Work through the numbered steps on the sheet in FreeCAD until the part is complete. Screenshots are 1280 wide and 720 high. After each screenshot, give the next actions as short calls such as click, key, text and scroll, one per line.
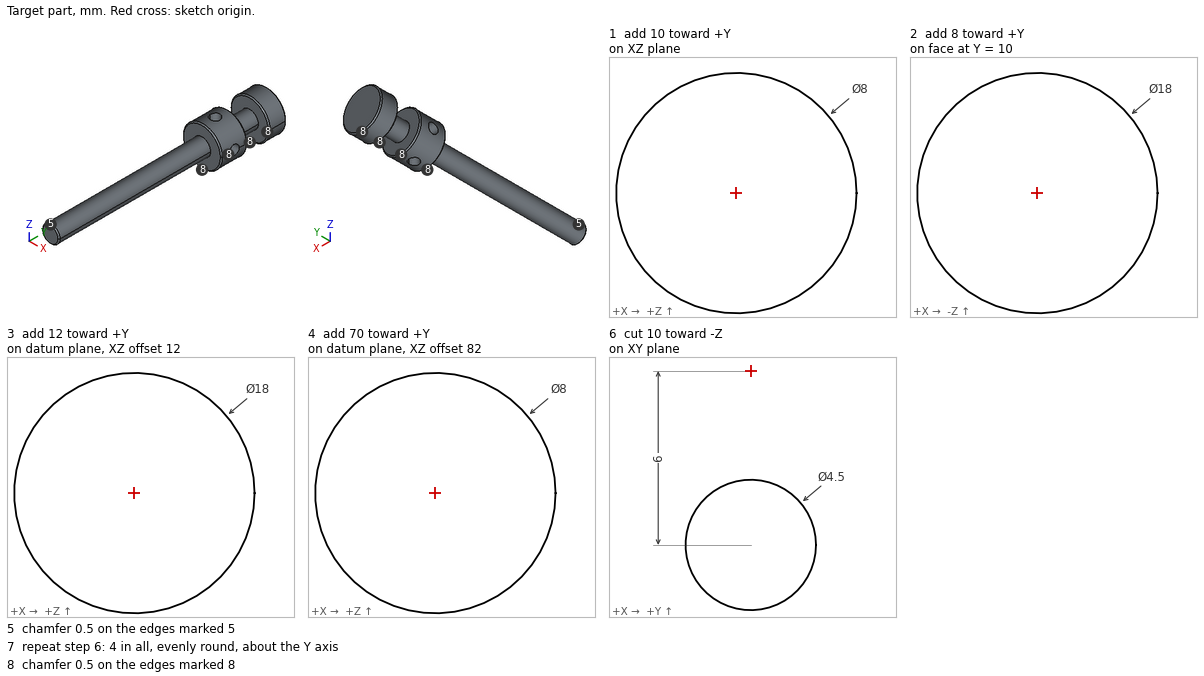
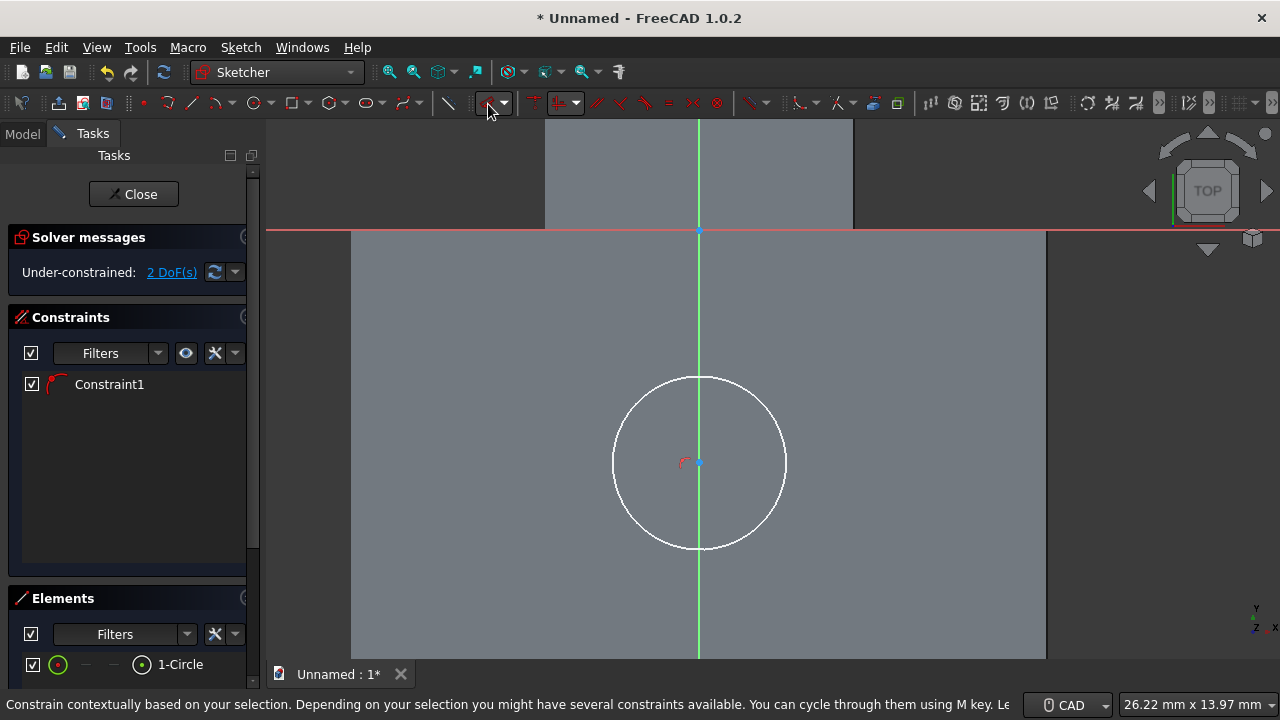
click(761, 402)
click(784, 379)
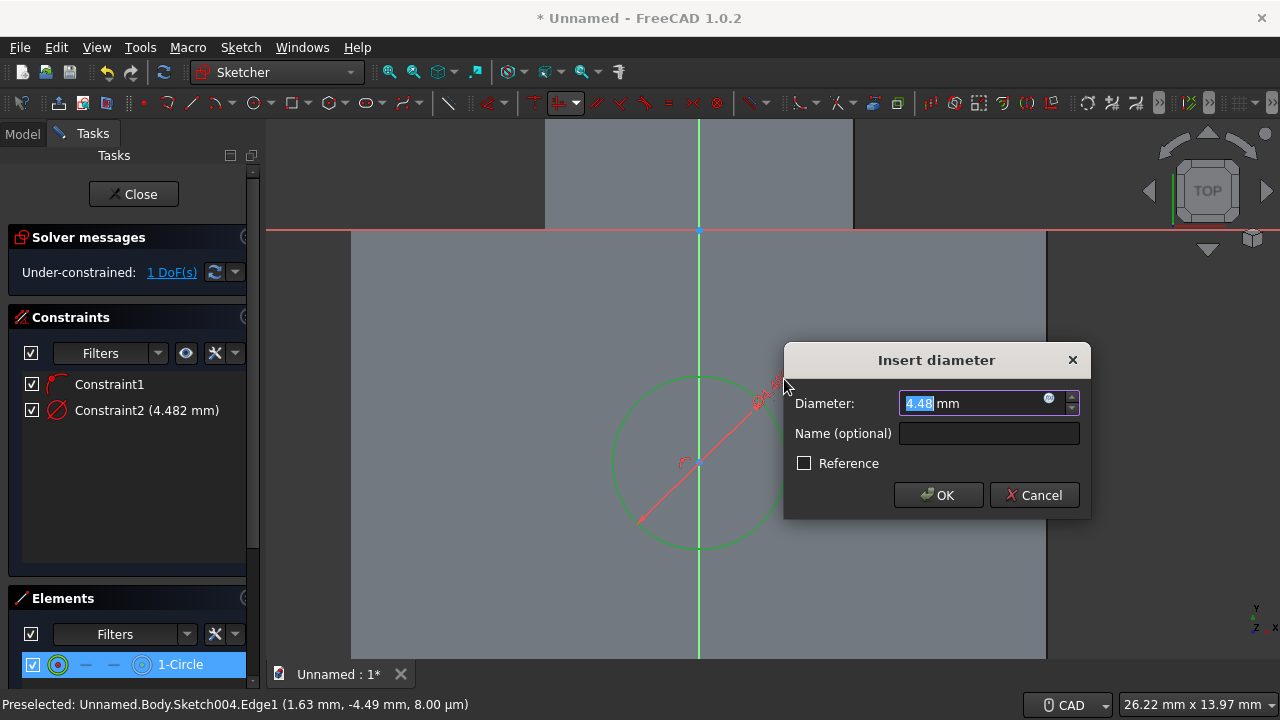
text(4.5)
key(Return)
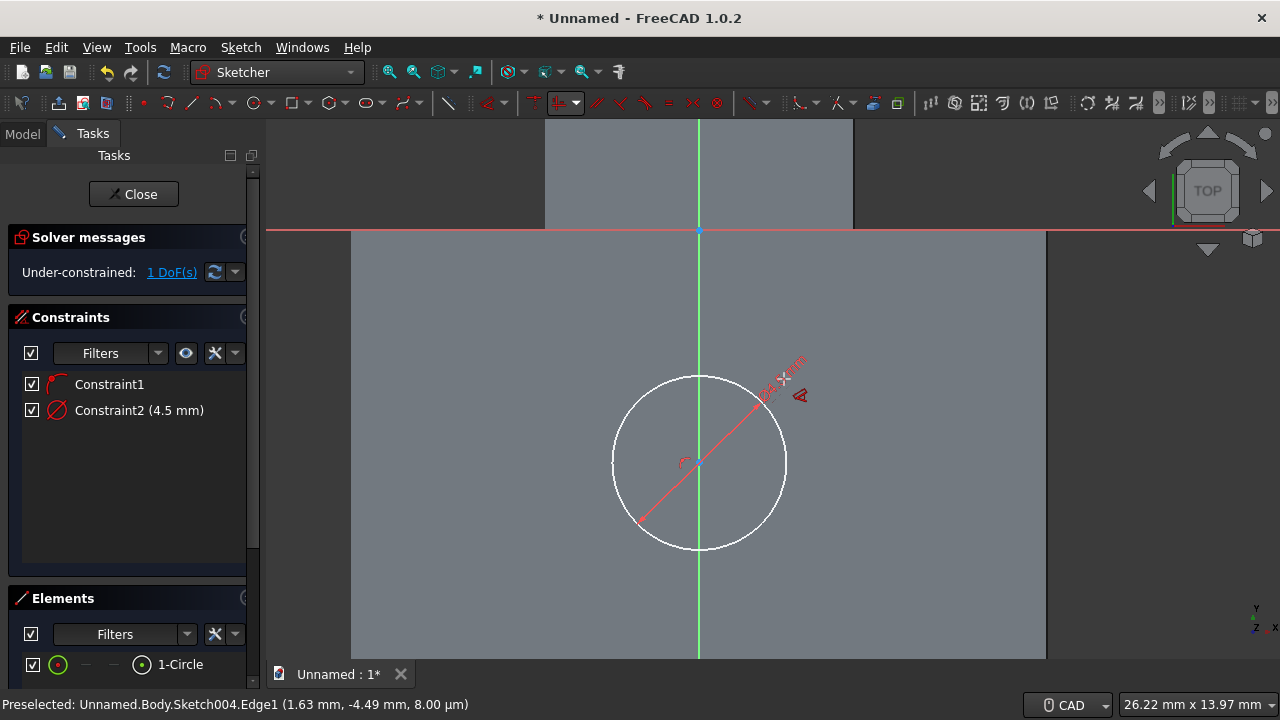
click(699, 463)
click(733, 347)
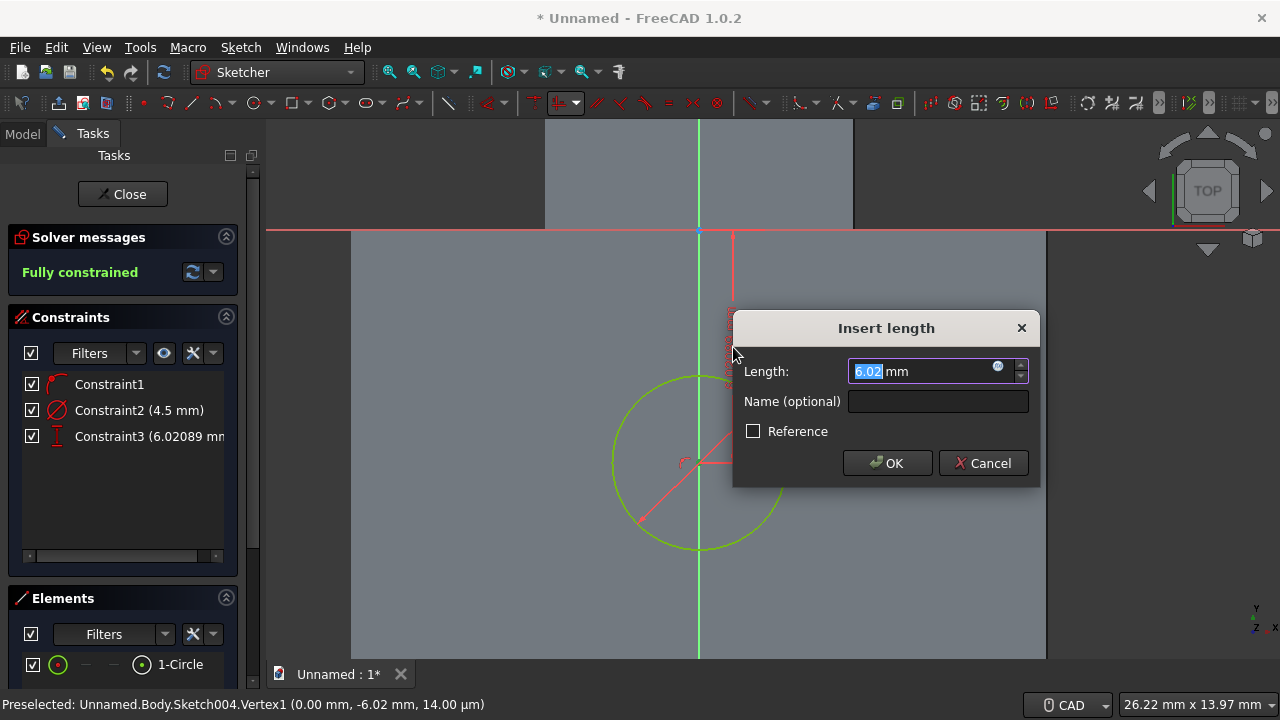
text(6)
key(Return)
key(Escape)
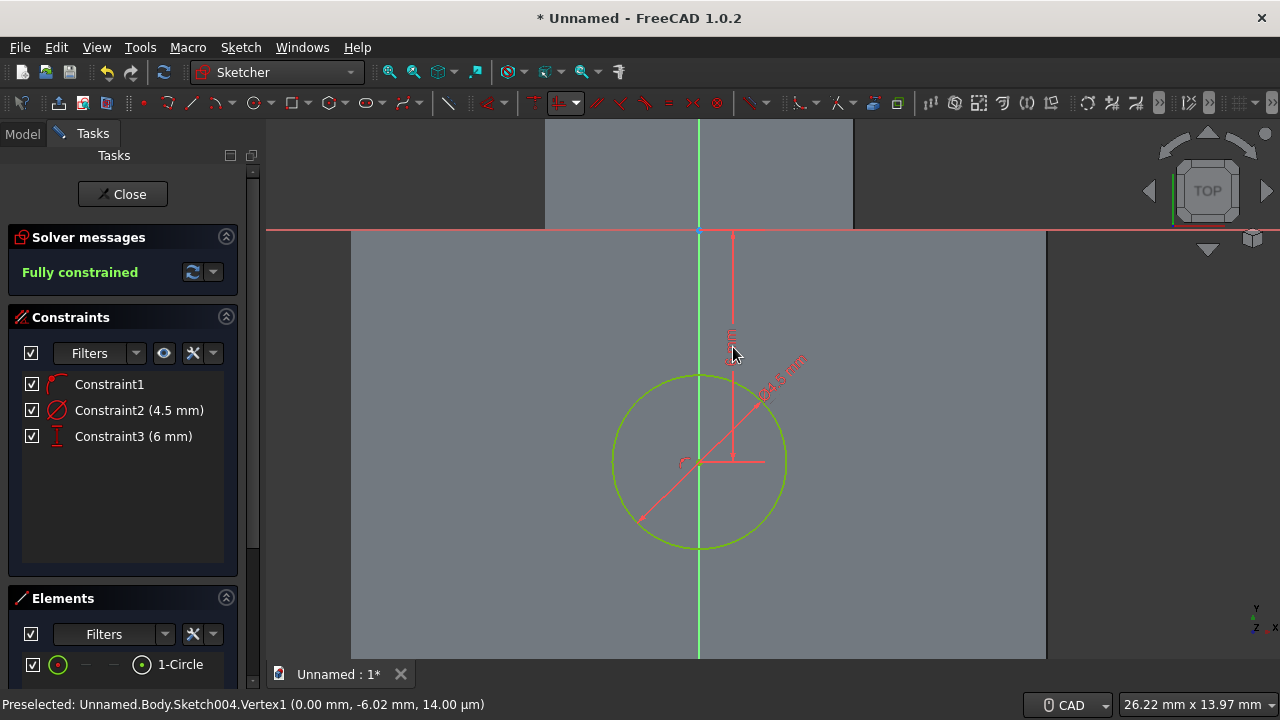
click(123, 194)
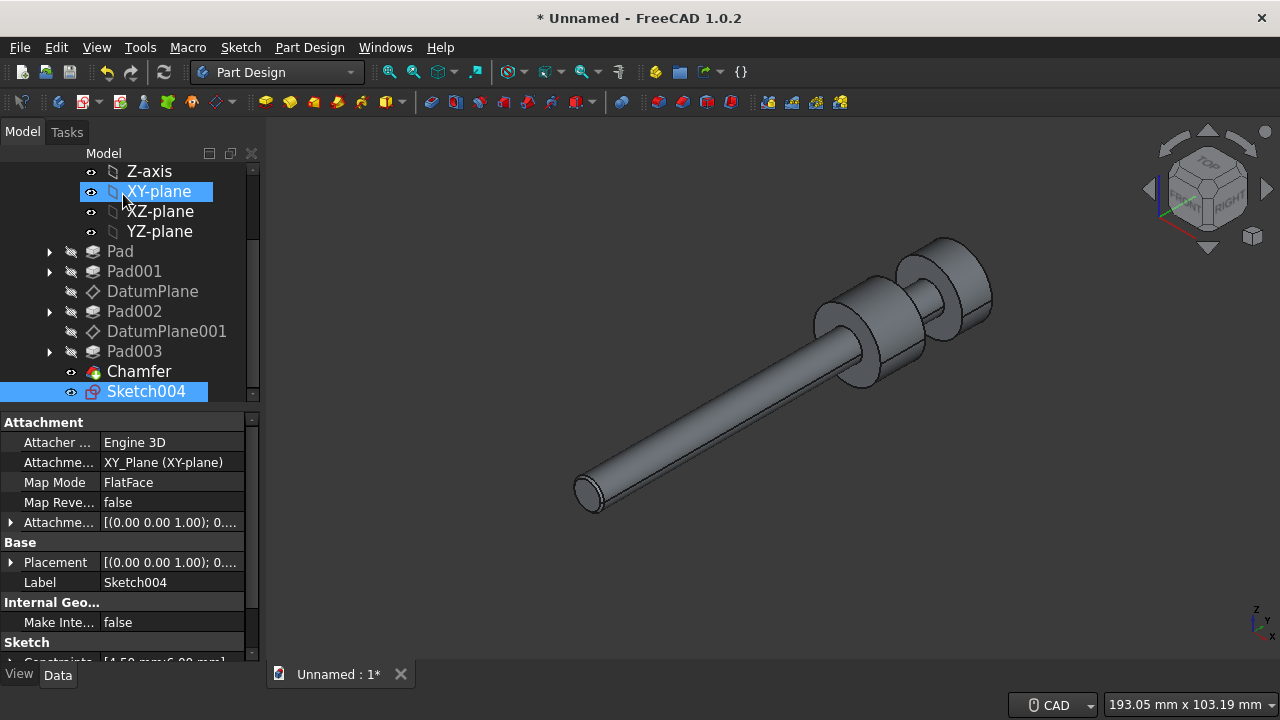
click(432, 102)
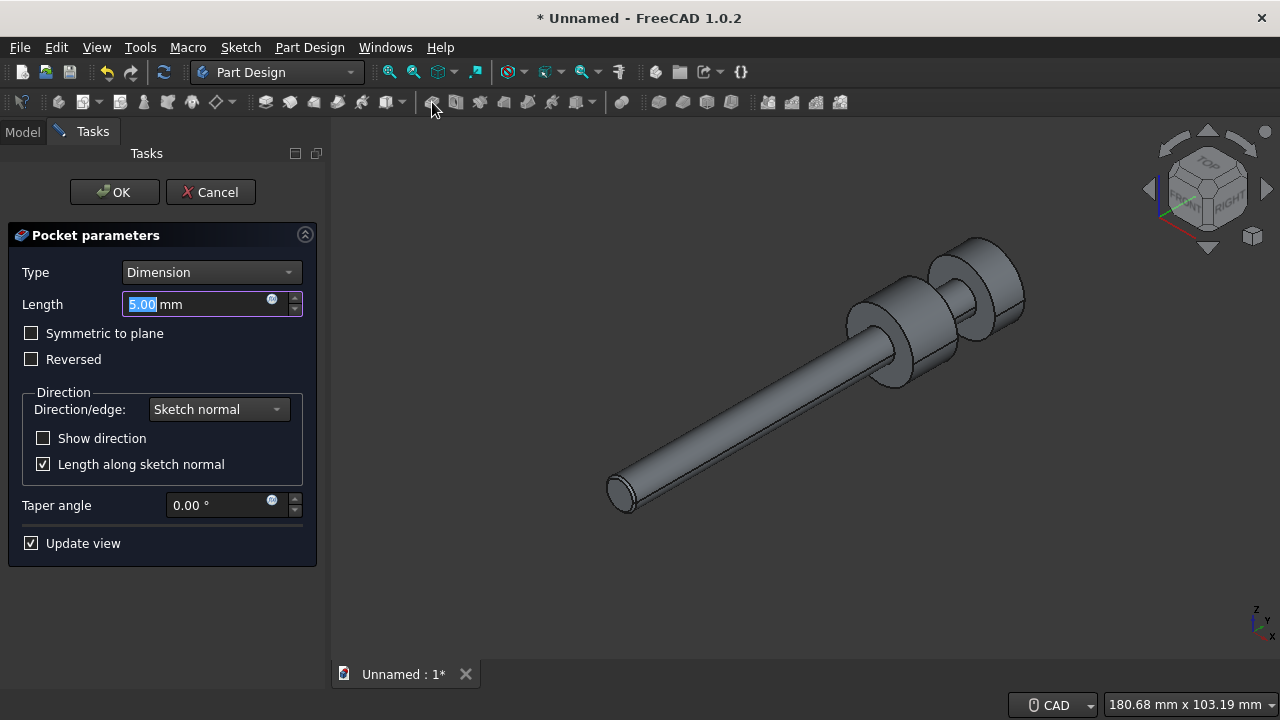
text(10)
key(Tab)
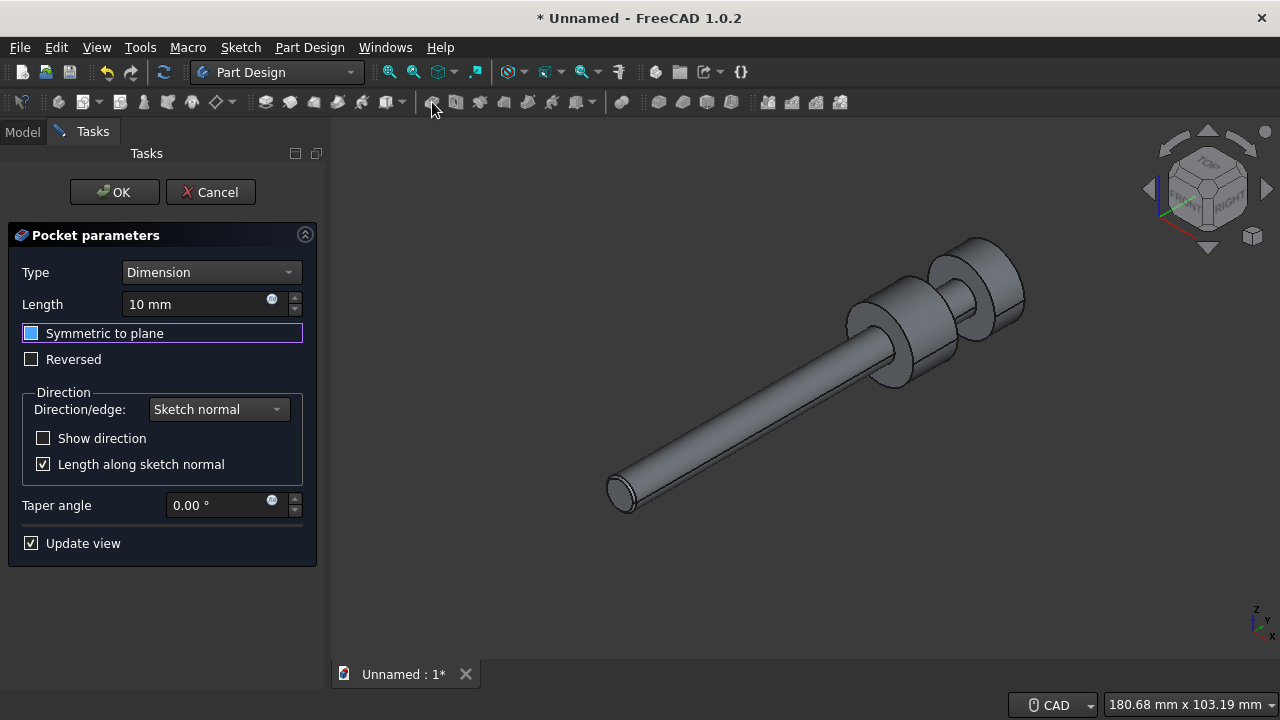
click(115, 192)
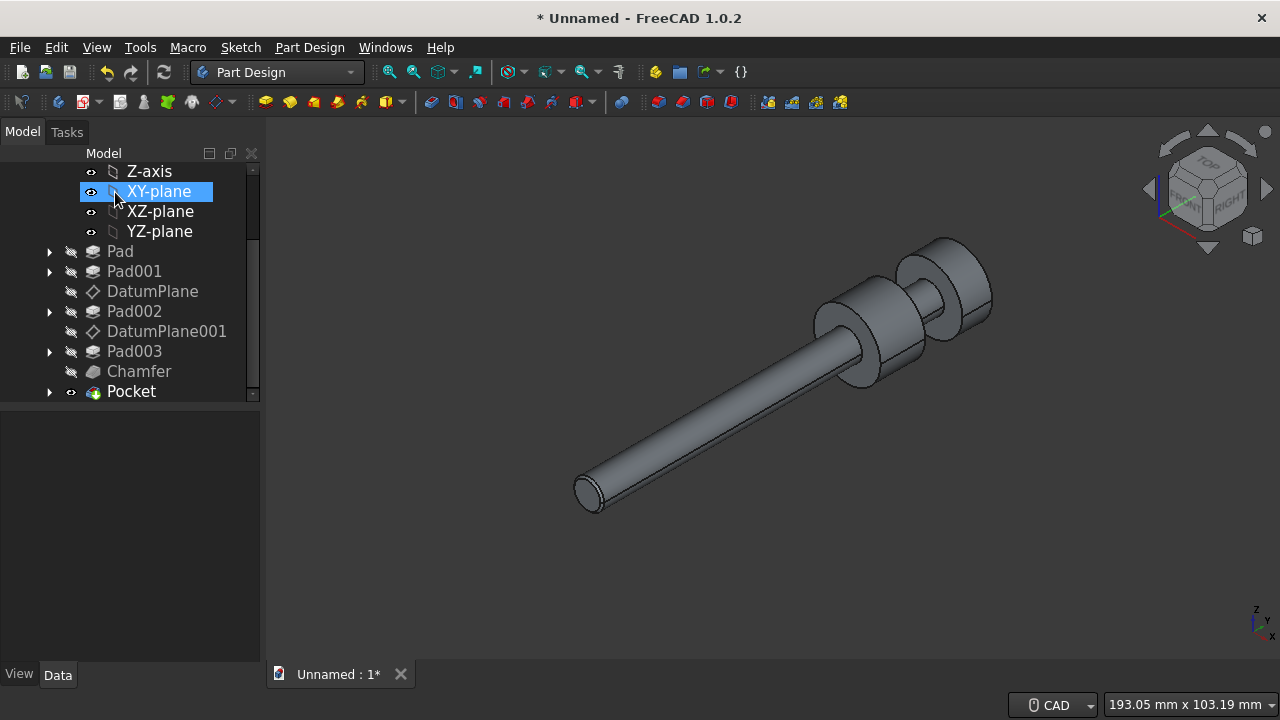
click(116, 392)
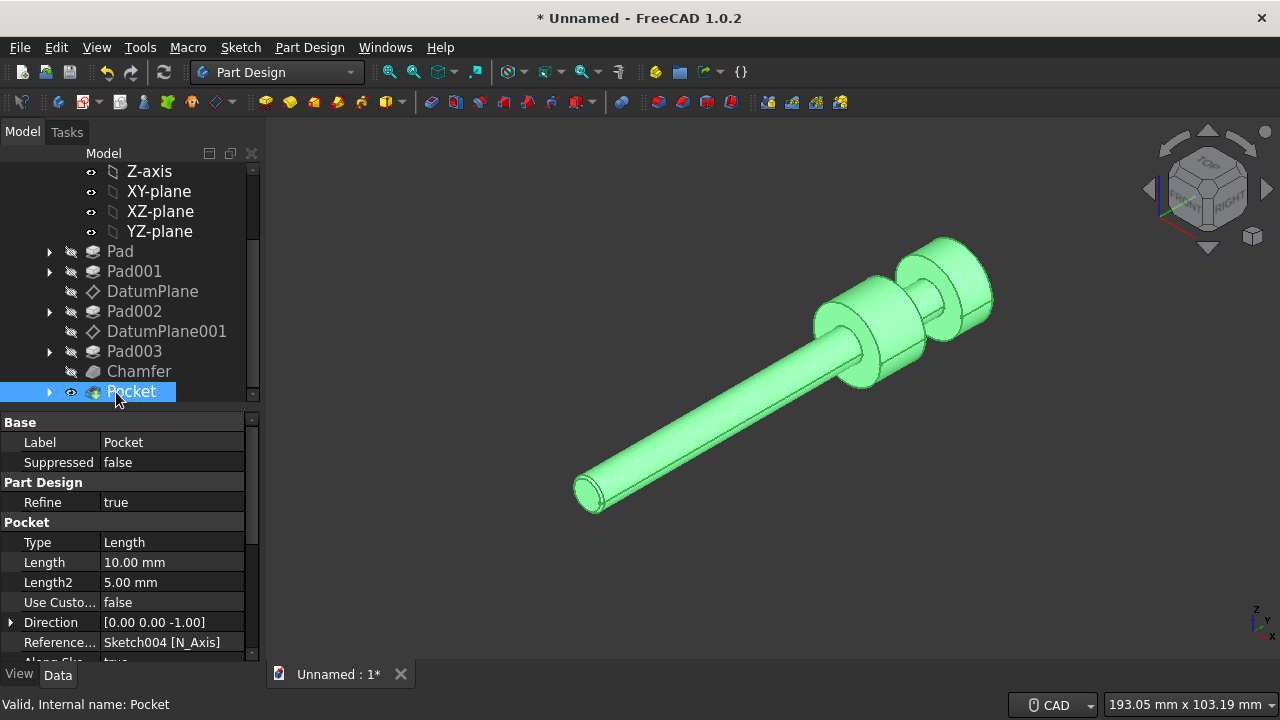
click(816, 102)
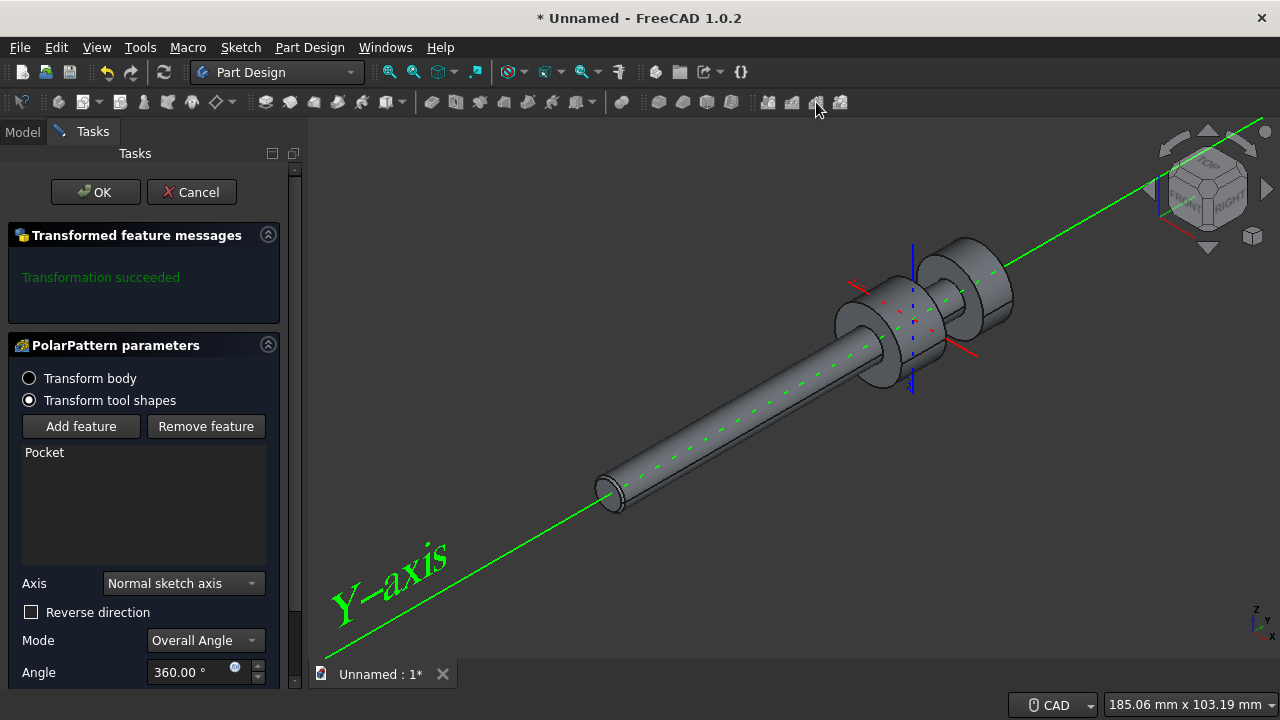
click(184, 584)